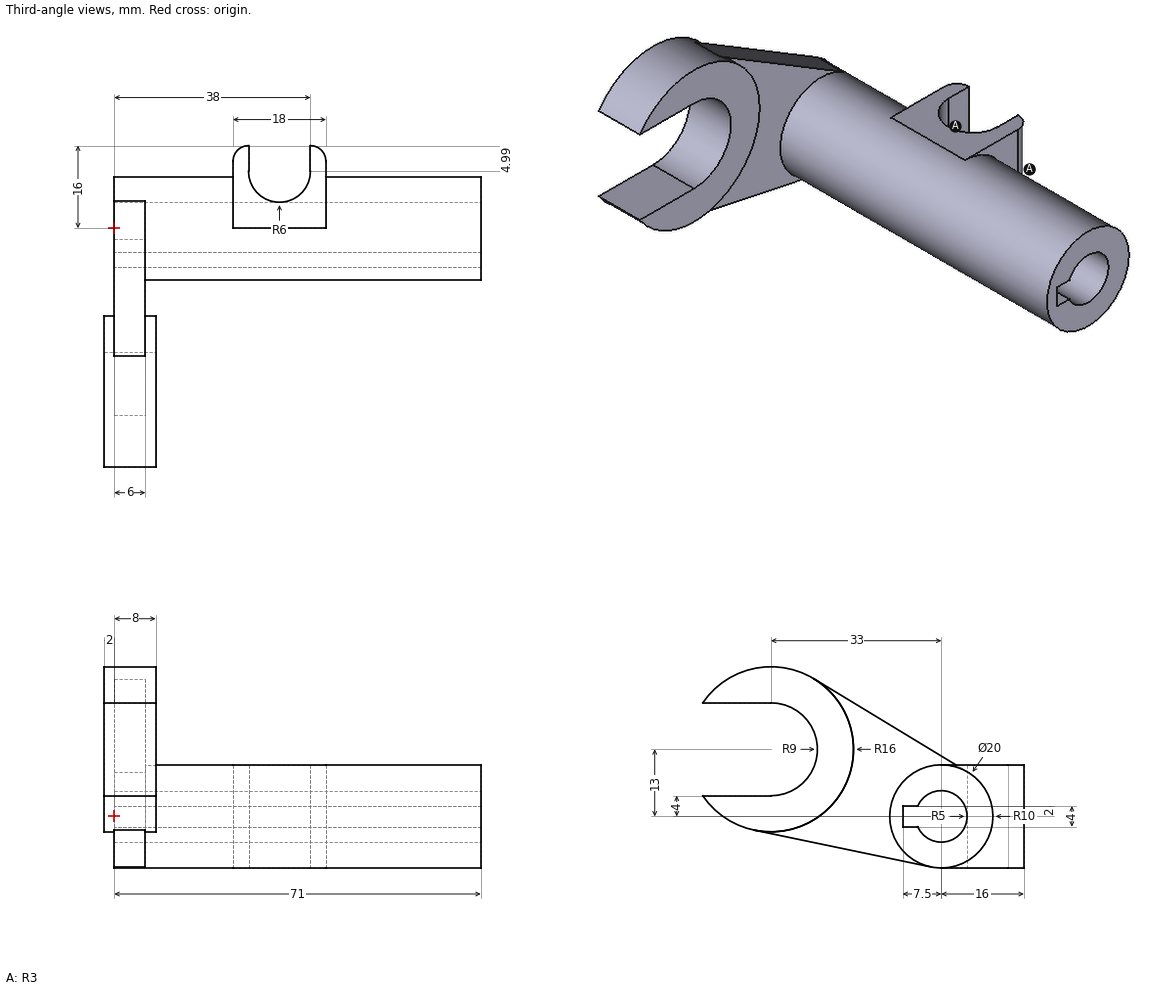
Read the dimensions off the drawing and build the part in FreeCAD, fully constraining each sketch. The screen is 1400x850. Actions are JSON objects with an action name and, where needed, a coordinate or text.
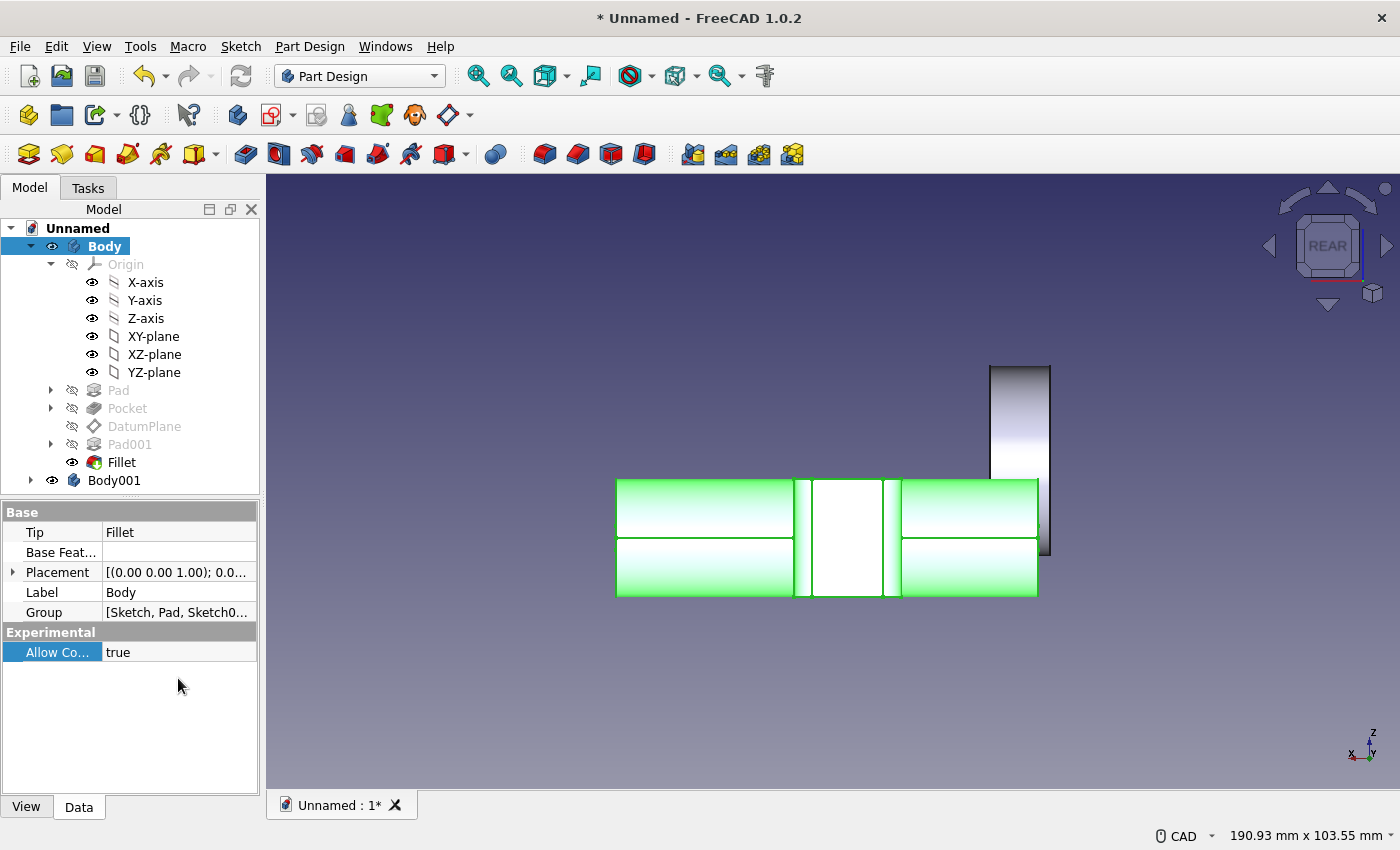
{"action": "left_click", "coordinate": [97, 480]}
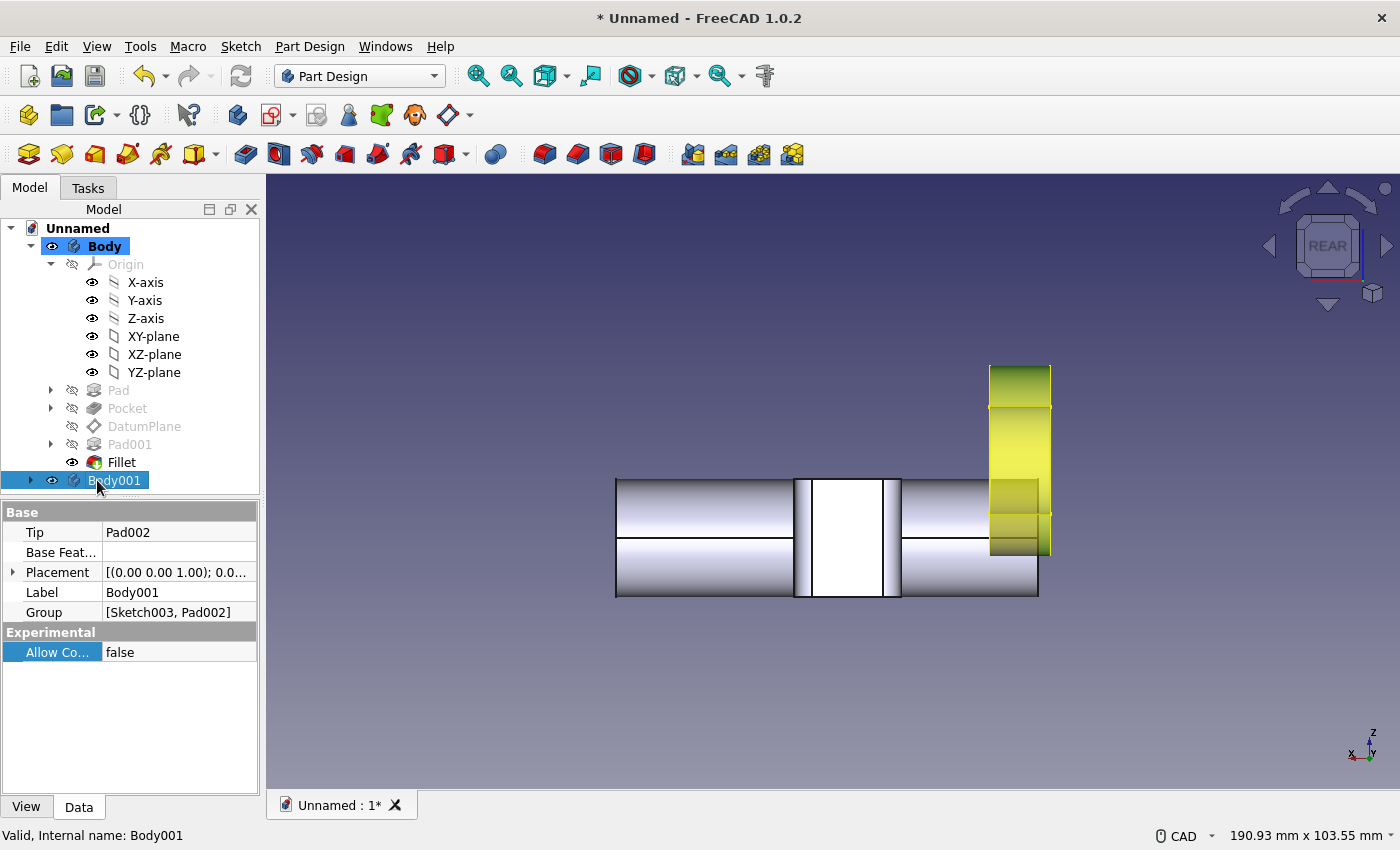
{"action": "left_click", "coordinate": [496, 154]}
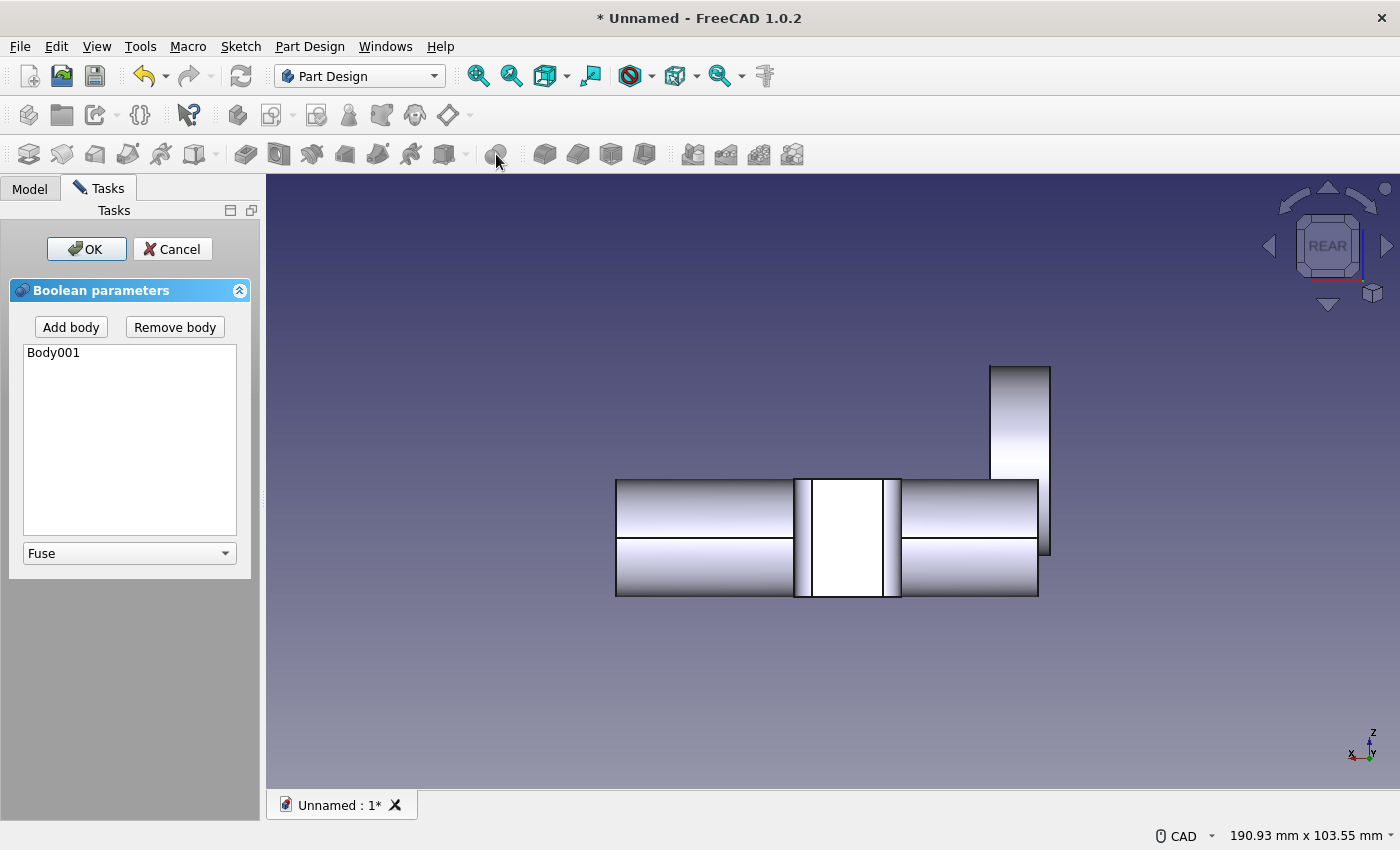
{"action": "left_click", "coordinate": [87, 249]}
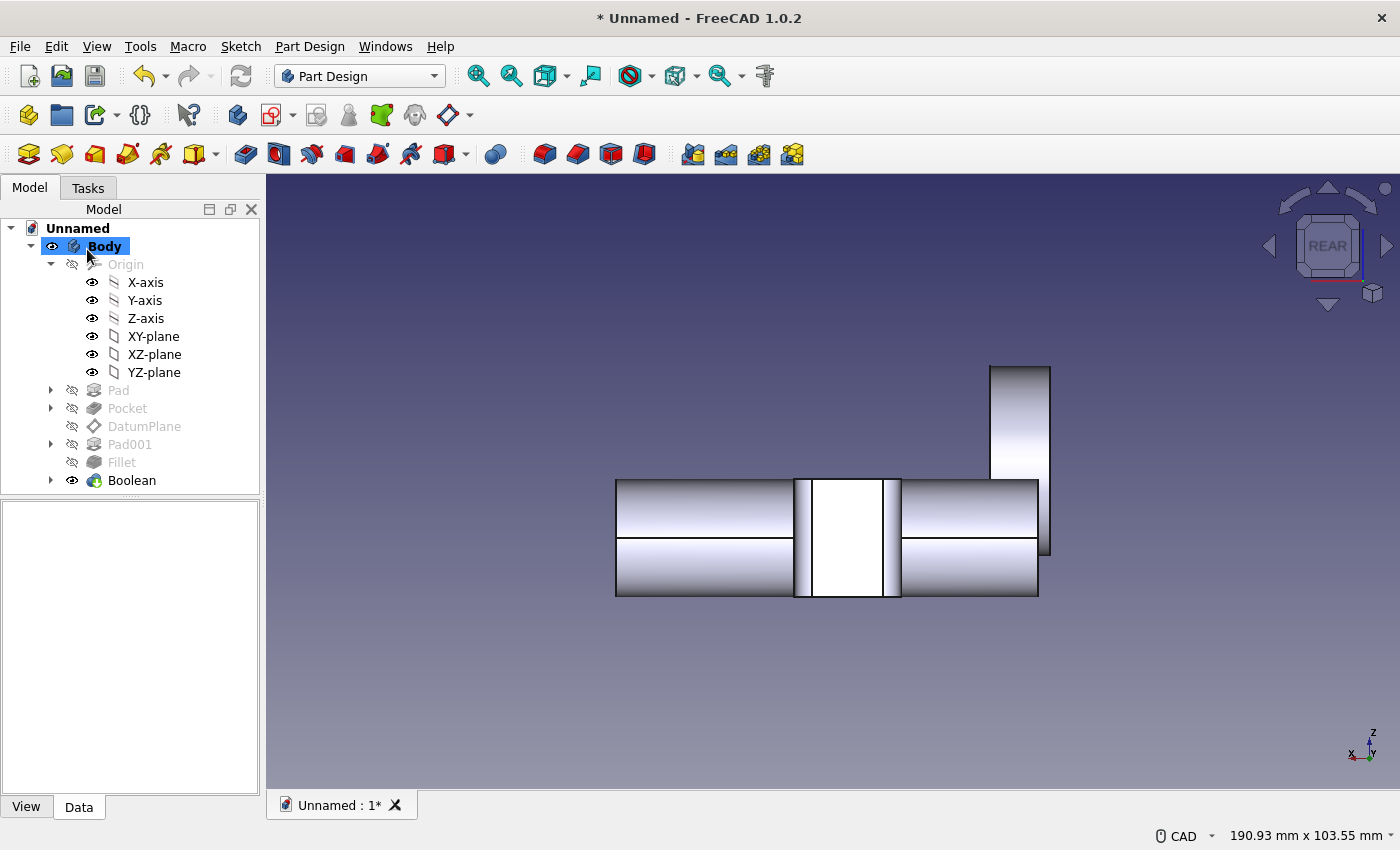
{"action": "key", "text": "v f"}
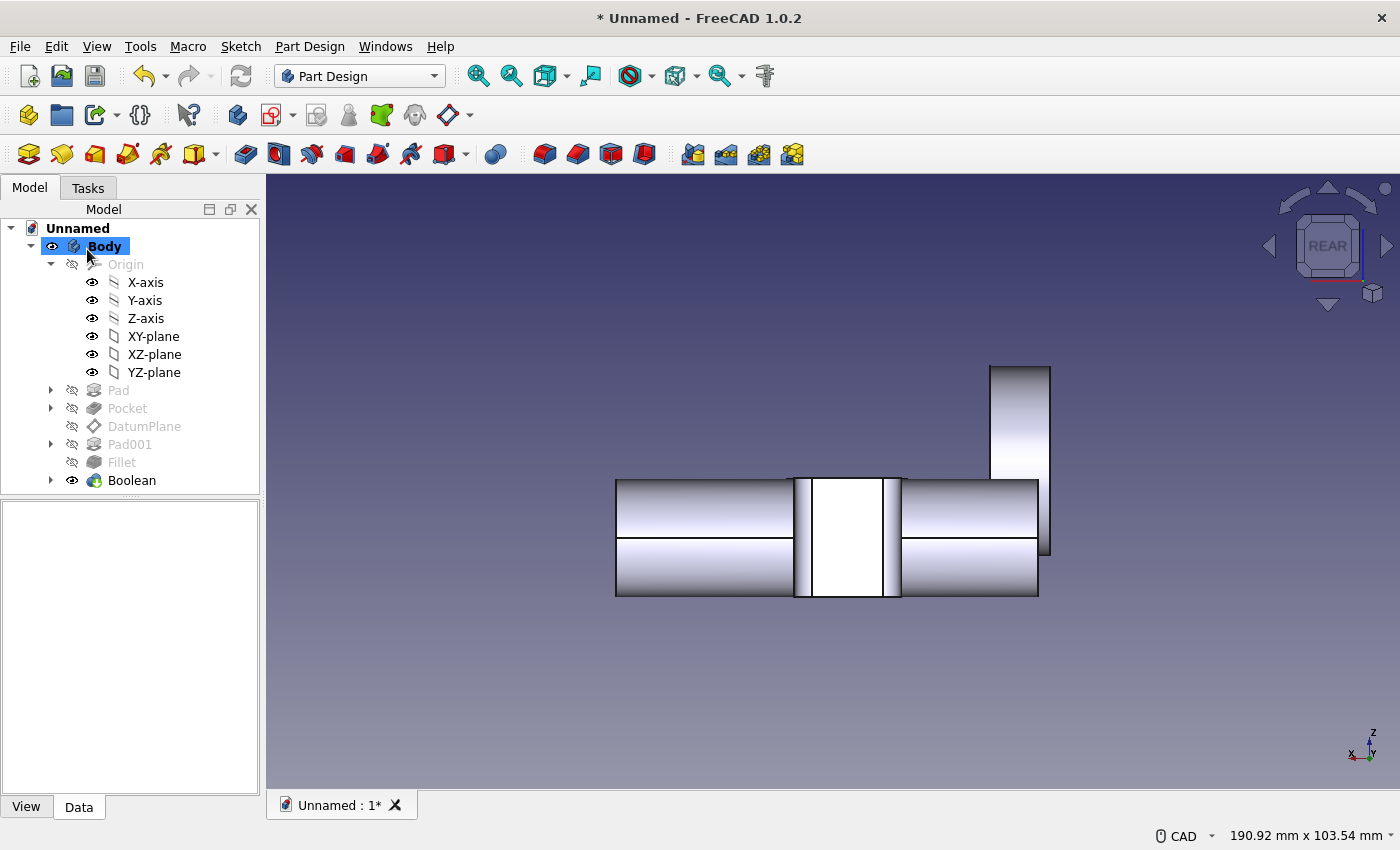
{"action": "left_click", "coordinate": [270, 116]}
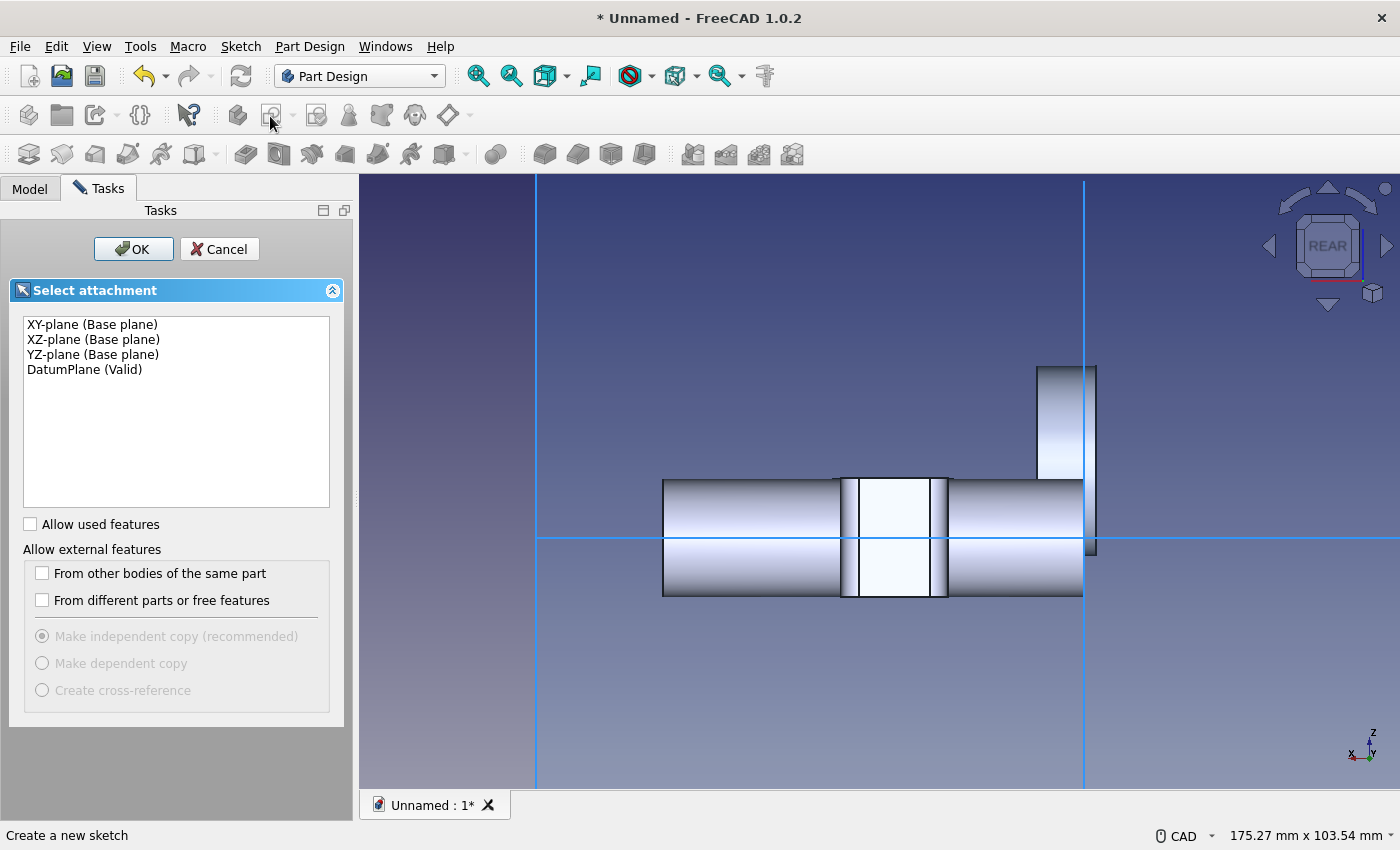
{"action": "left_click", "coordinate": [84, 354]}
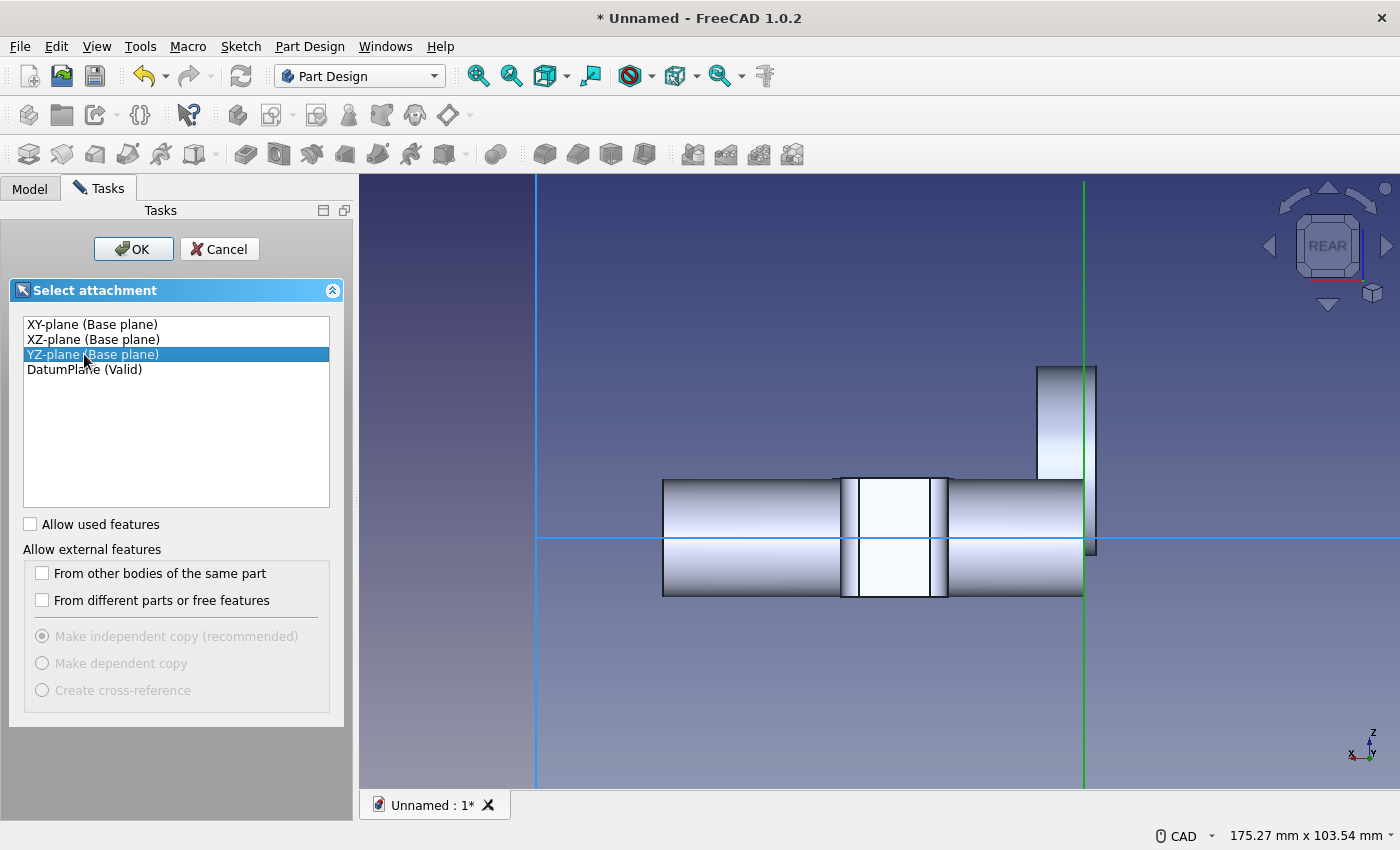
{"action": "left_click", "coordinate": [134, 249]}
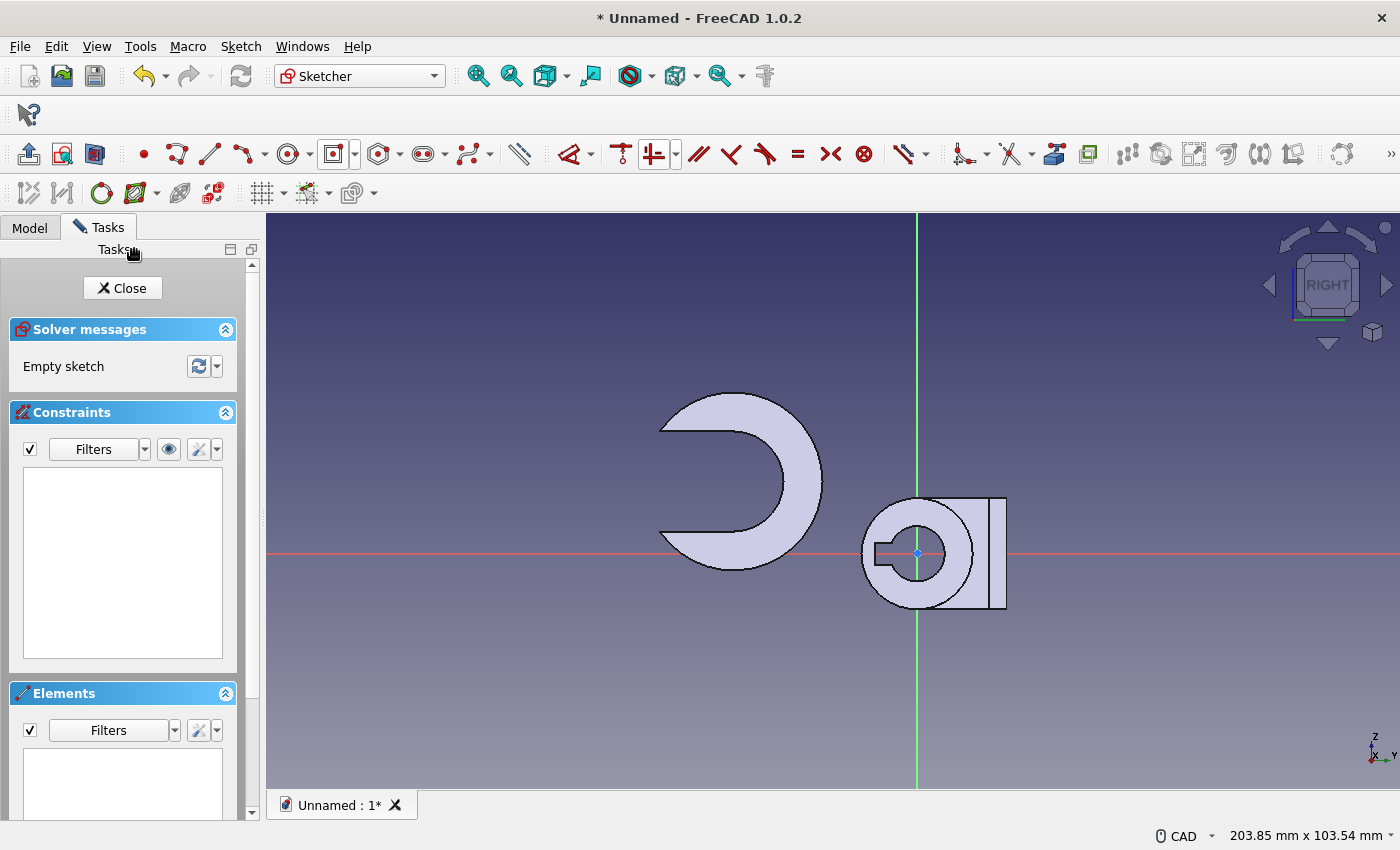
{"action": "left_click", "coordinate": [95, 154]}